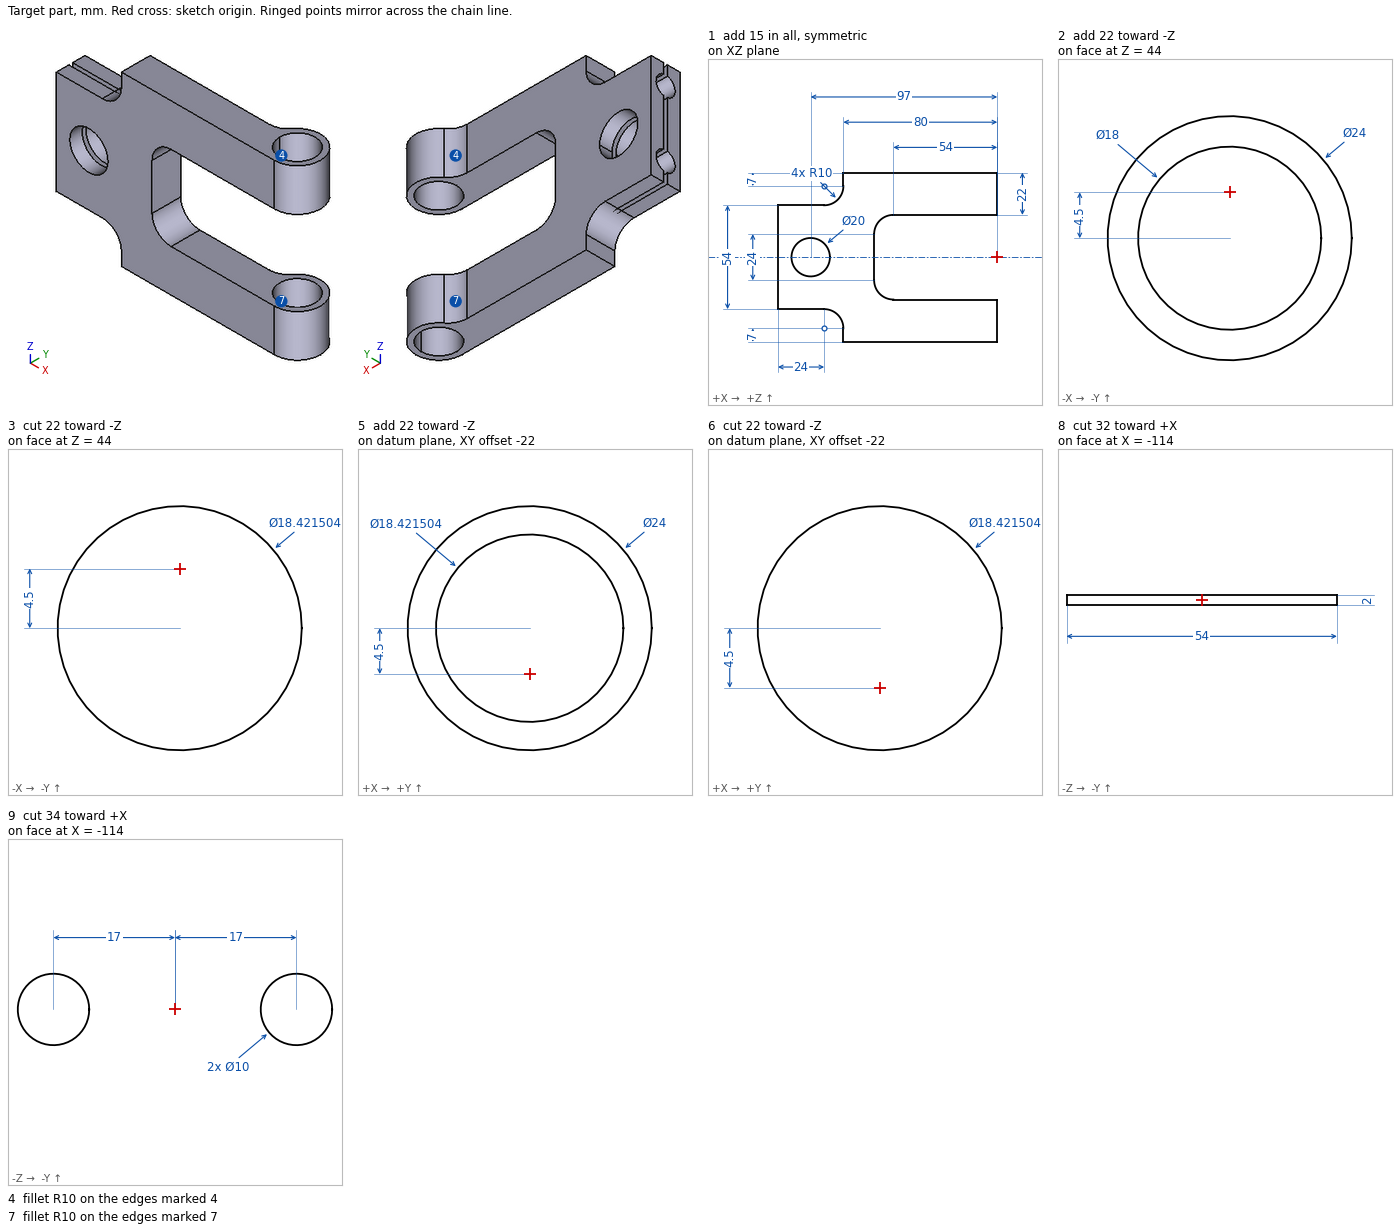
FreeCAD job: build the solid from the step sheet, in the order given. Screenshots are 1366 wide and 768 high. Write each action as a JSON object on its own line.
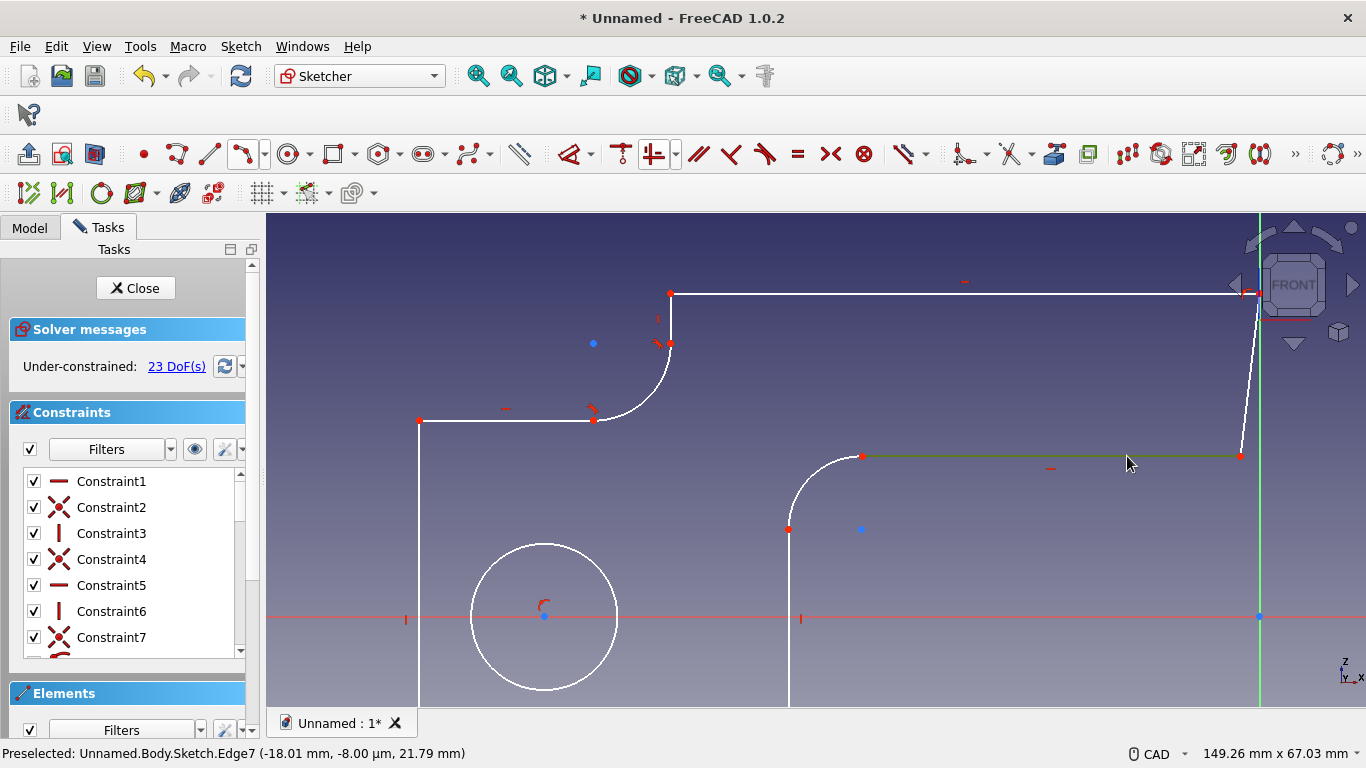
{"action": "left_click", "coordinate": [829, 464]}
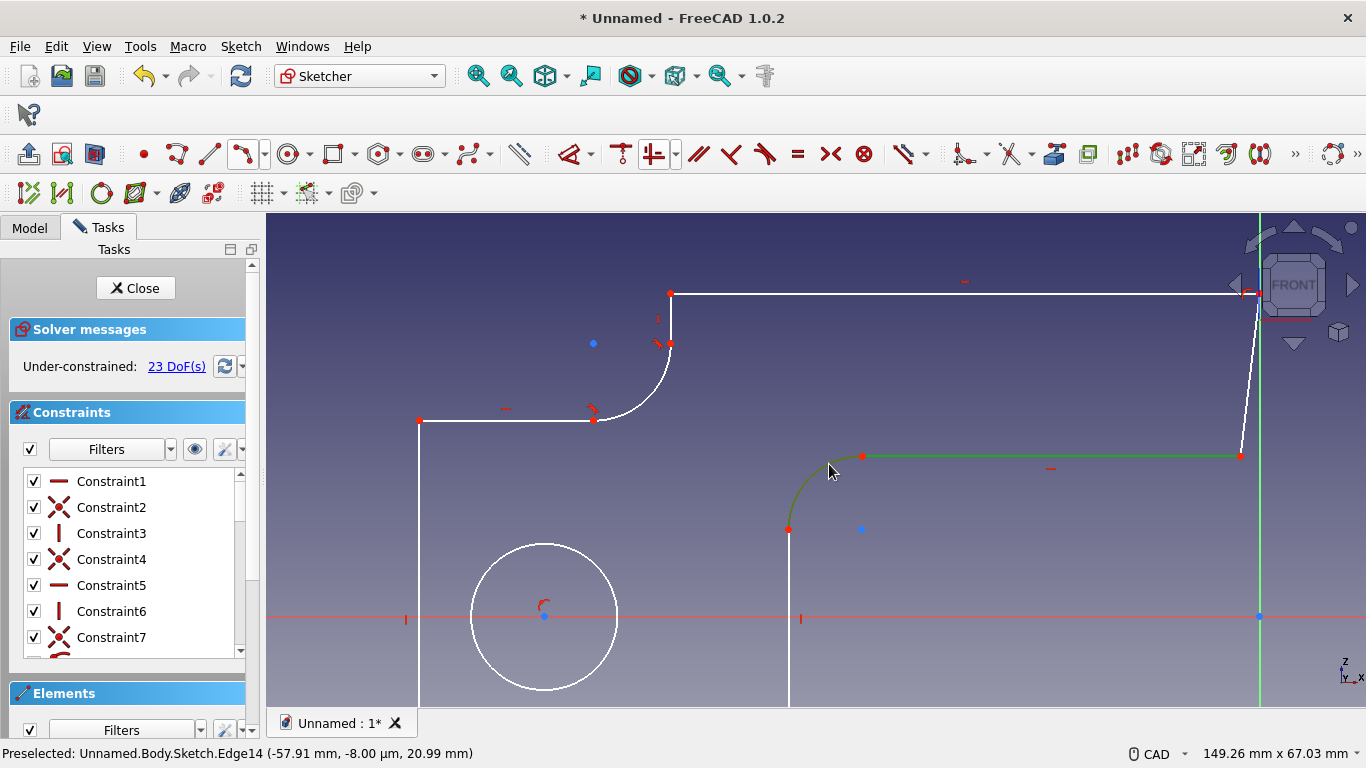
{"action": "left_click", "coordinate": [765, 154]}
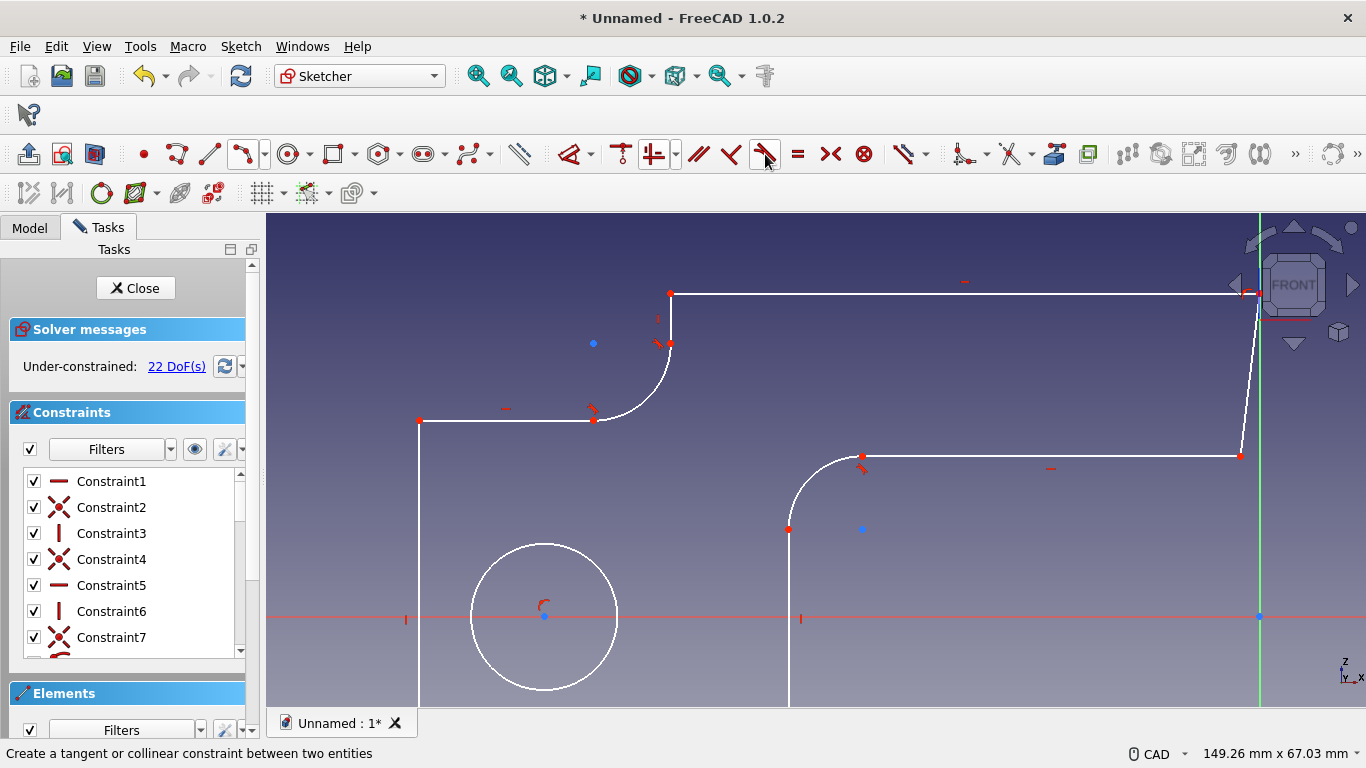
{"action": "left_click", "coordinate": [789, 583]}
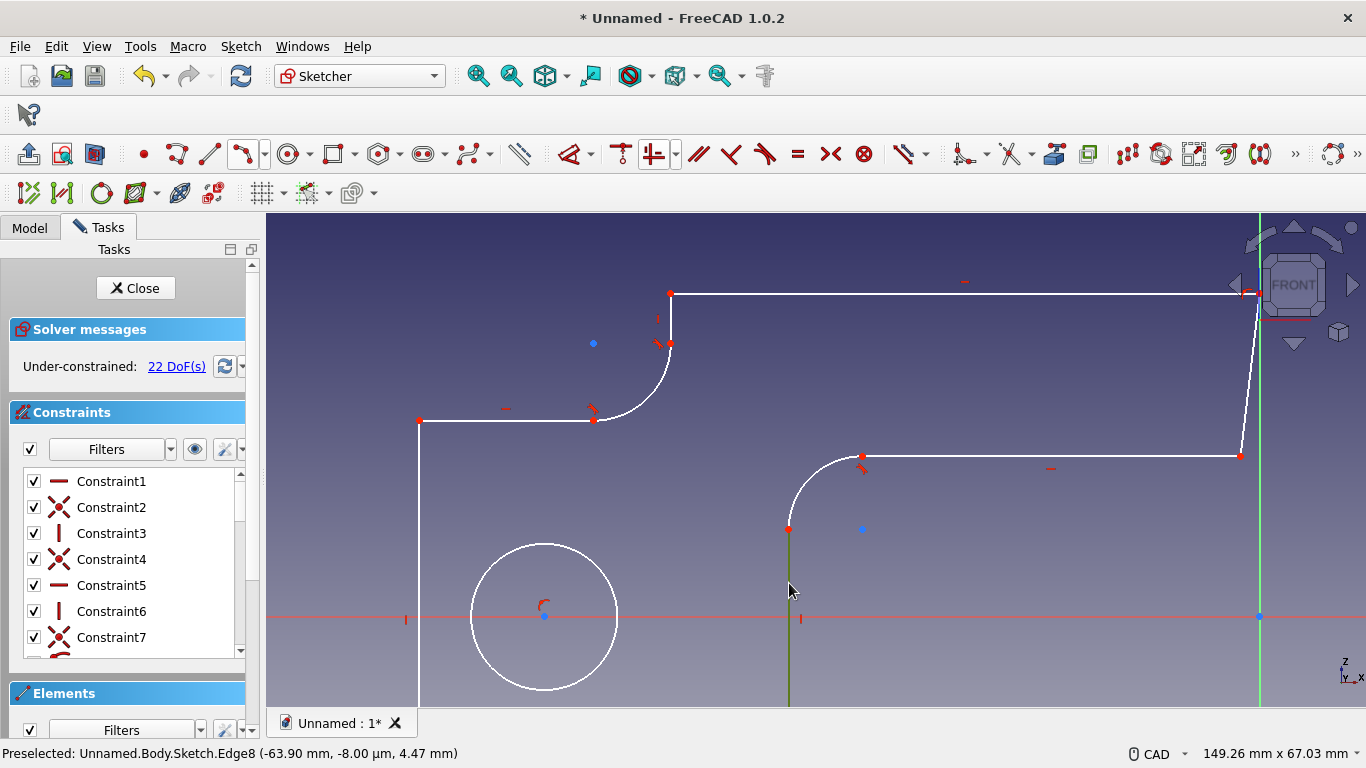
{"action": "left_click", "coordinate": [829, 464]}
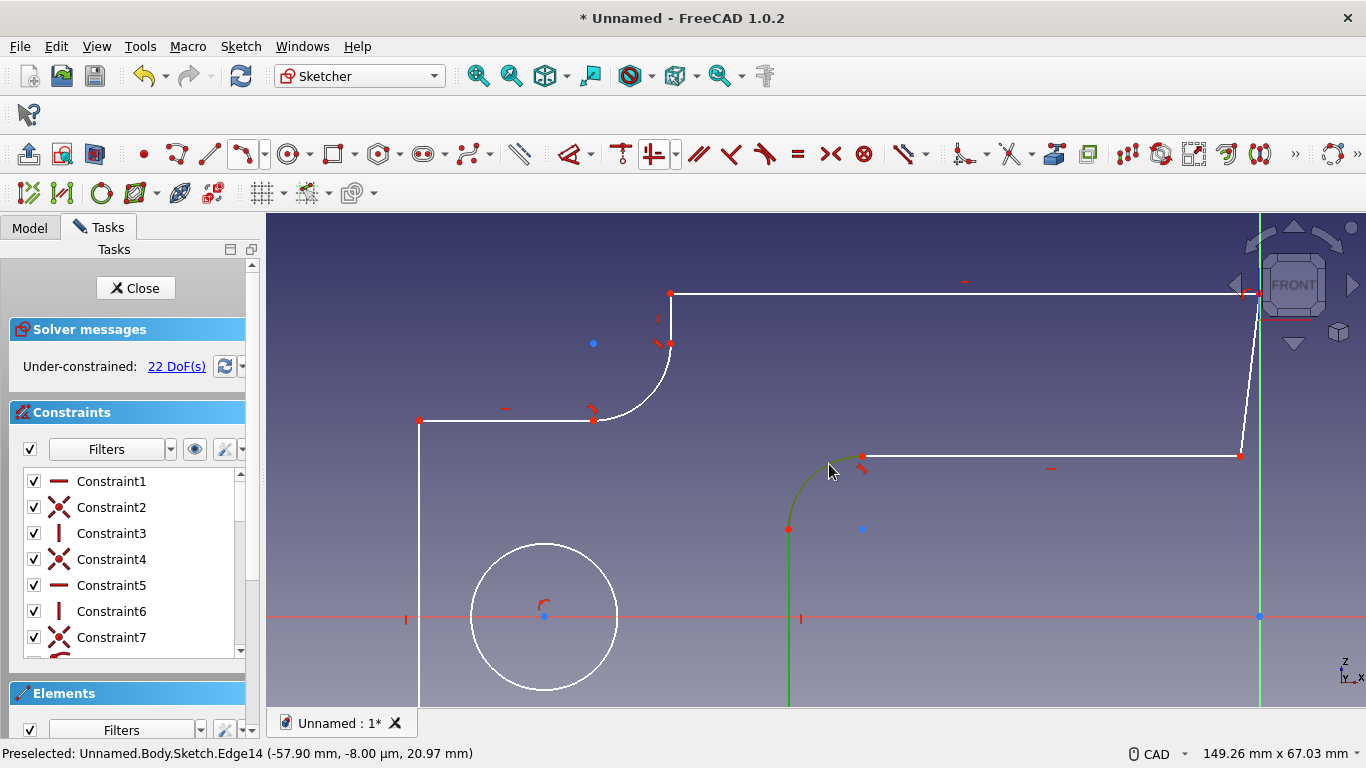
{"action": "left_click", "coordinate": [765, 154]}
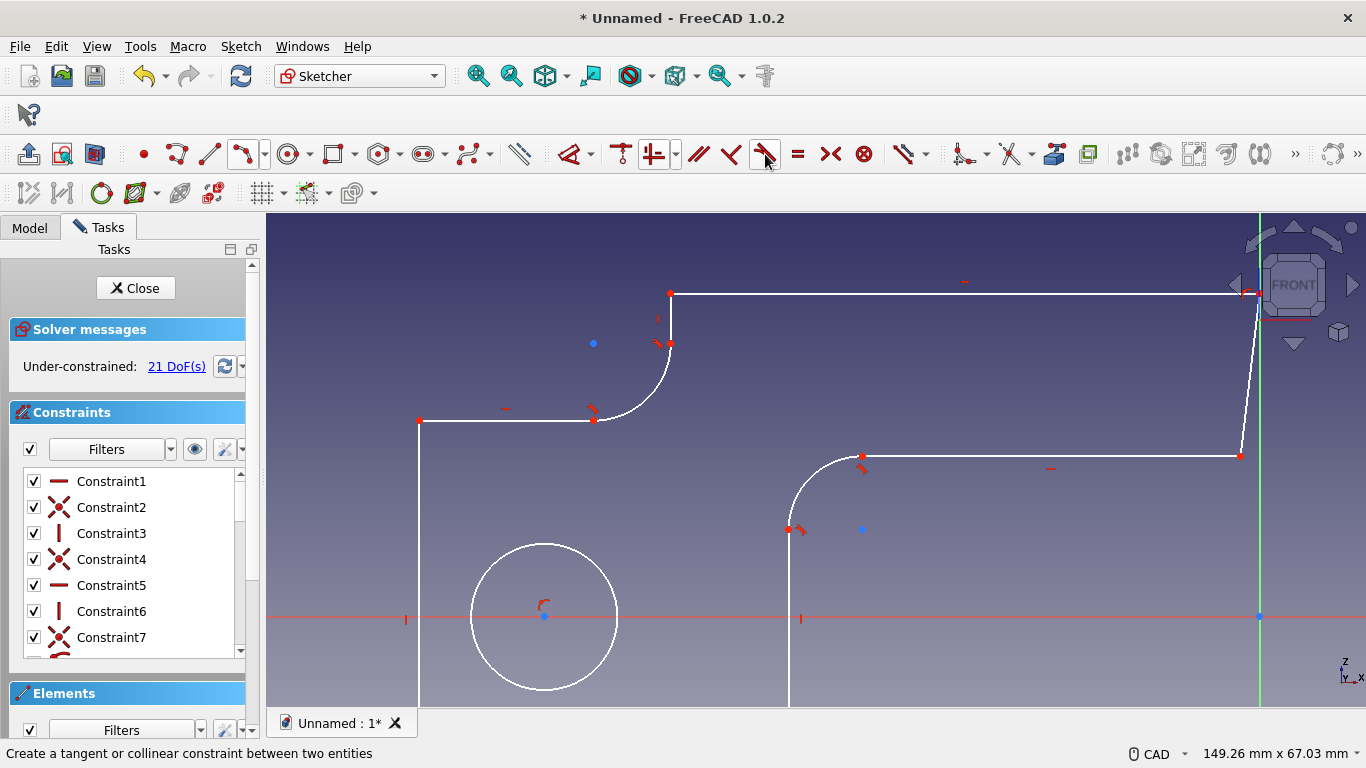
{"action": "left_click", "coordinate": [789, 583]}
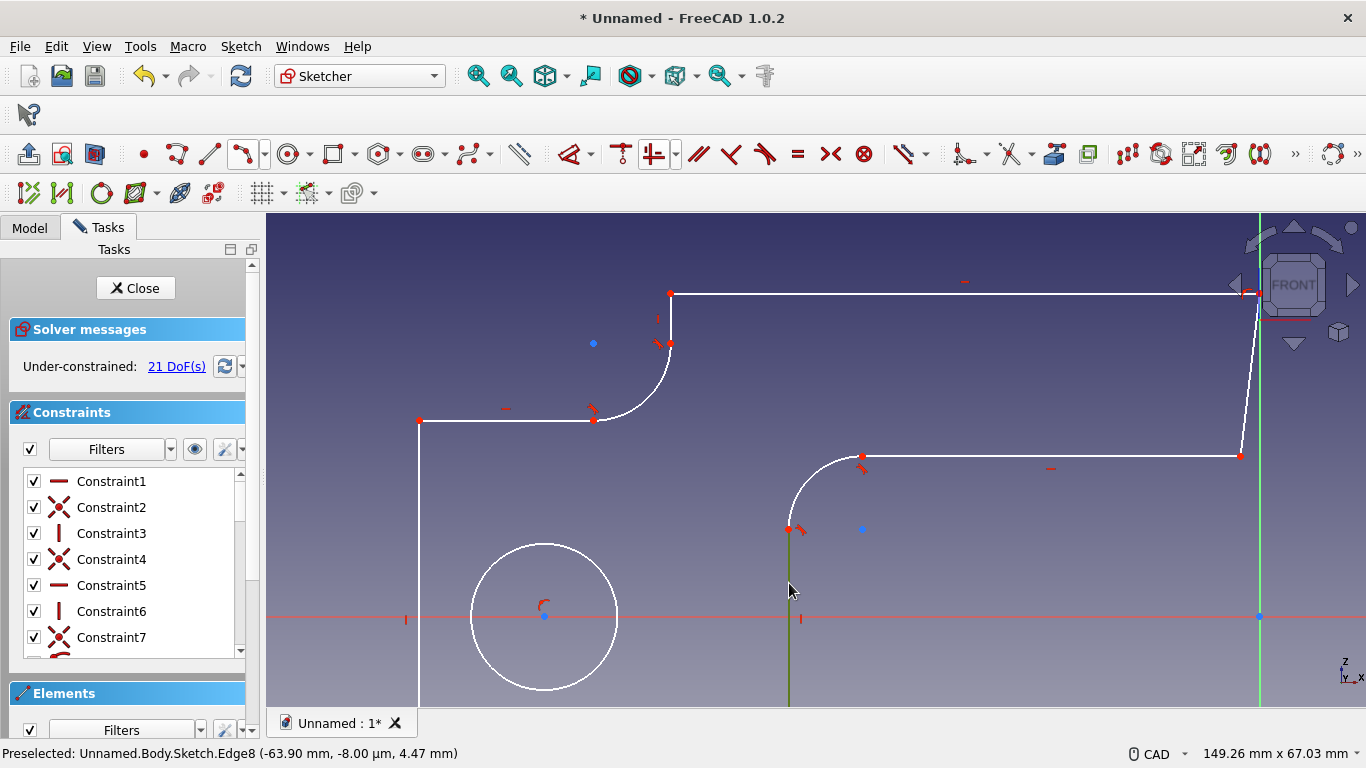
{"action": "scroll", "coordinate": [672, 332], "scroll_direction": "down", "scroll_amount": 4}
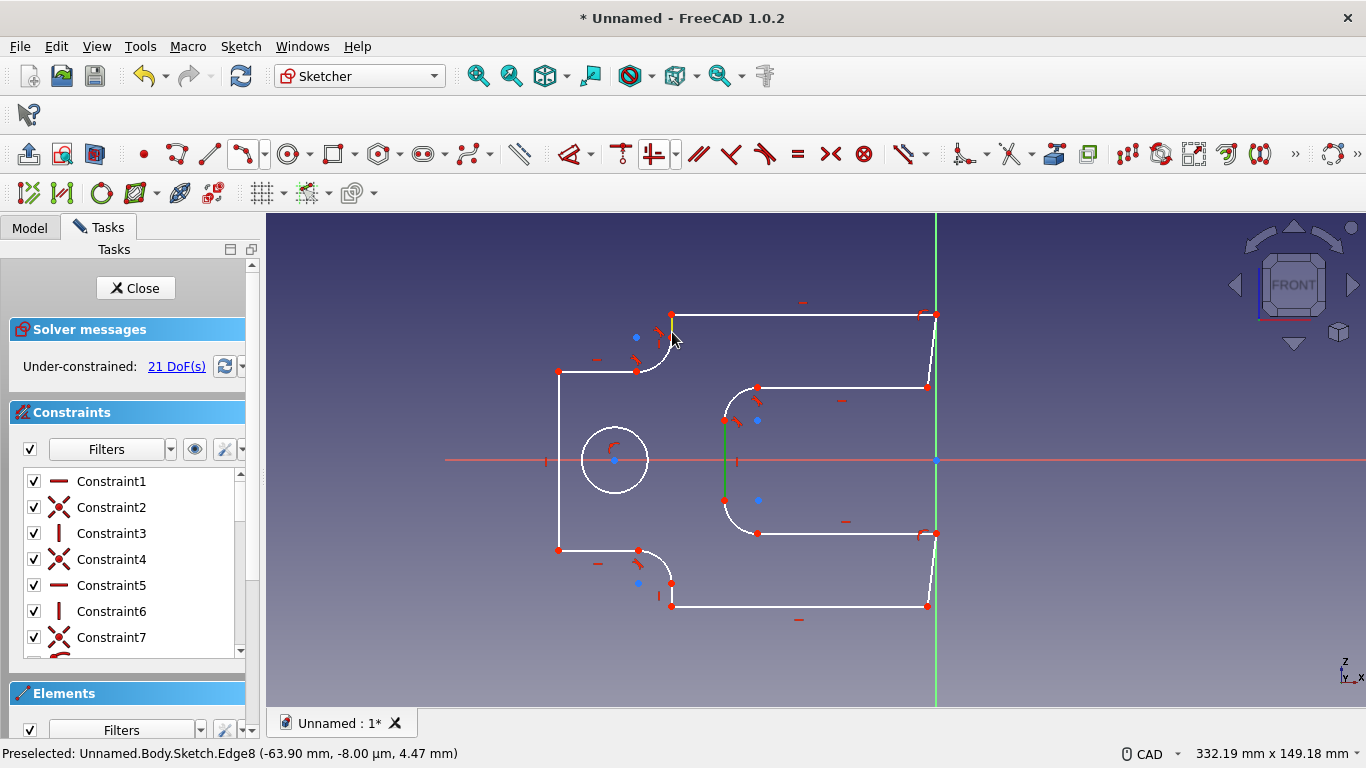
{"action": "left_click", "coordinate": [728, 516]}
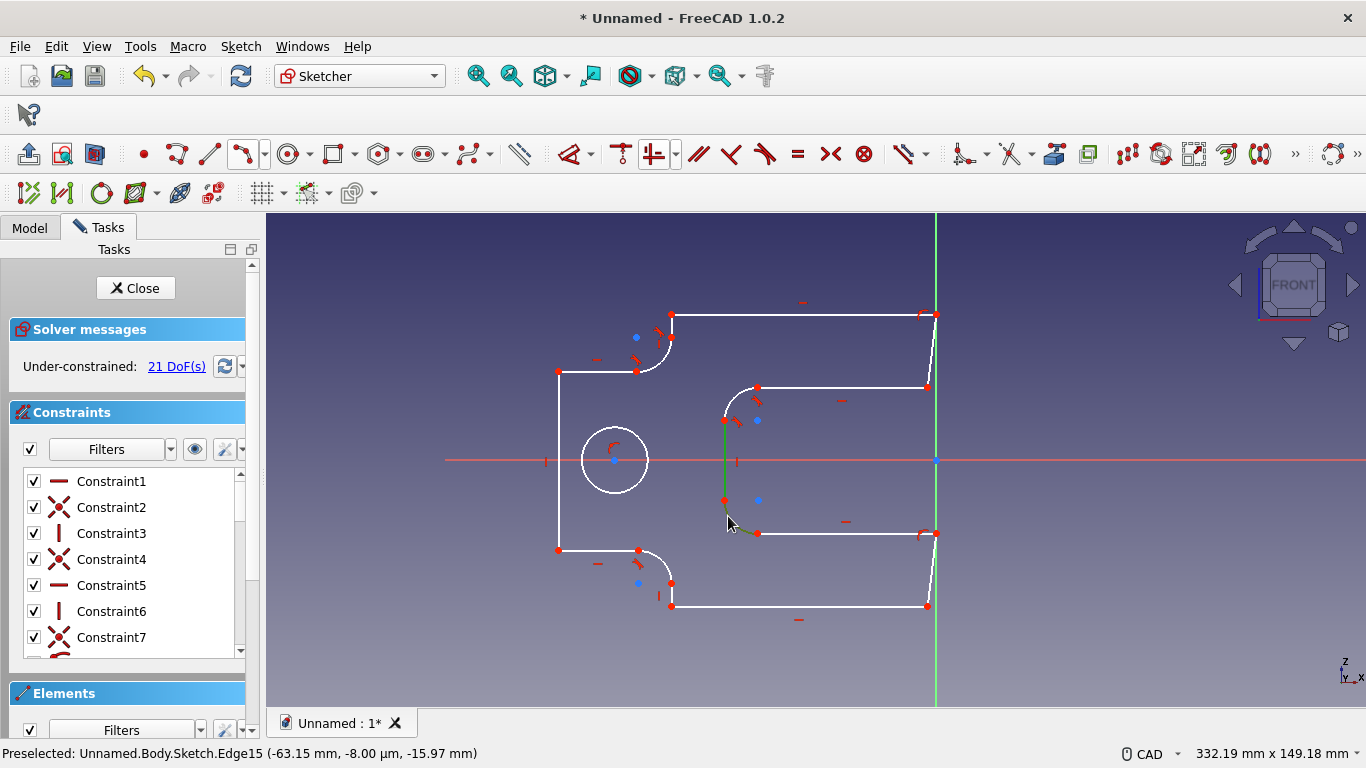
{"action": "left_click", "coordinate": [765, 154]}